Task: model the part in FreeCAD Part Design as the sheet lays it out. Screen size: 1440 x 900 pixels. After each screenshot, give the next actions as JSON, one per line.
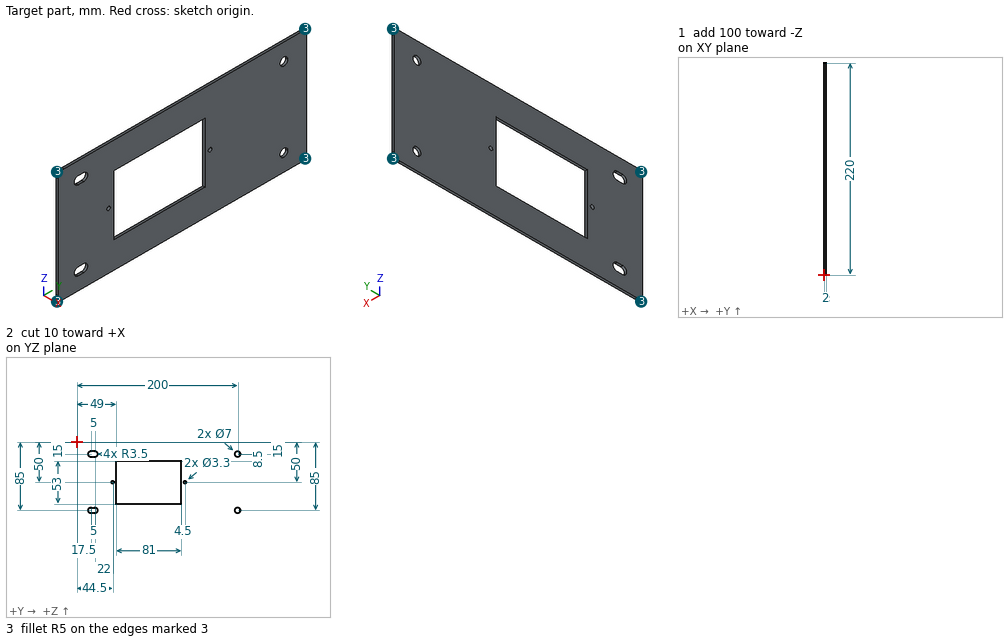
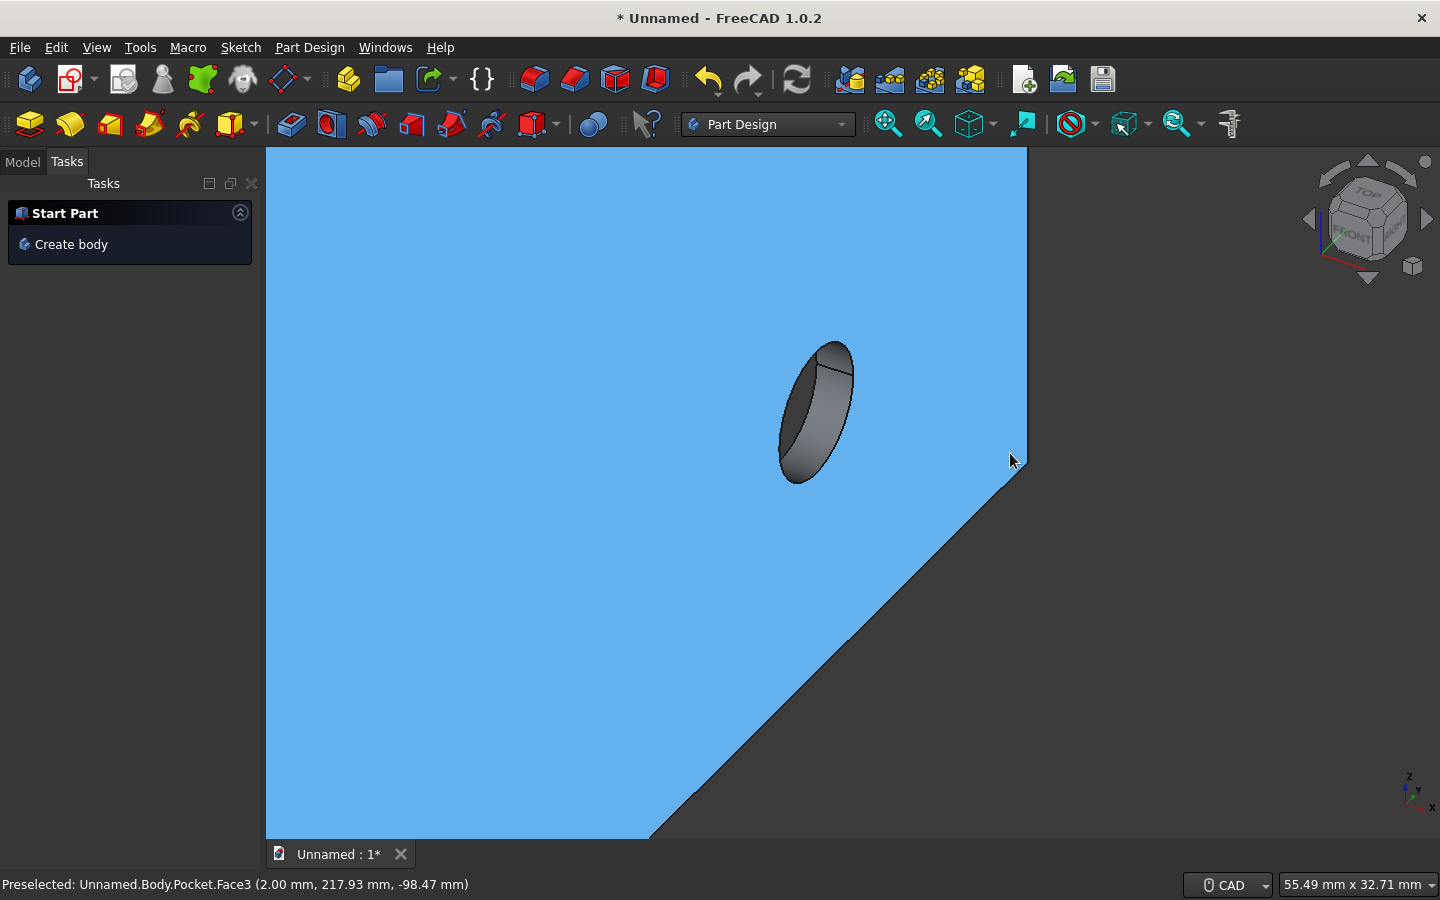
{"action": "left_click", "coordinate": [890, 124]}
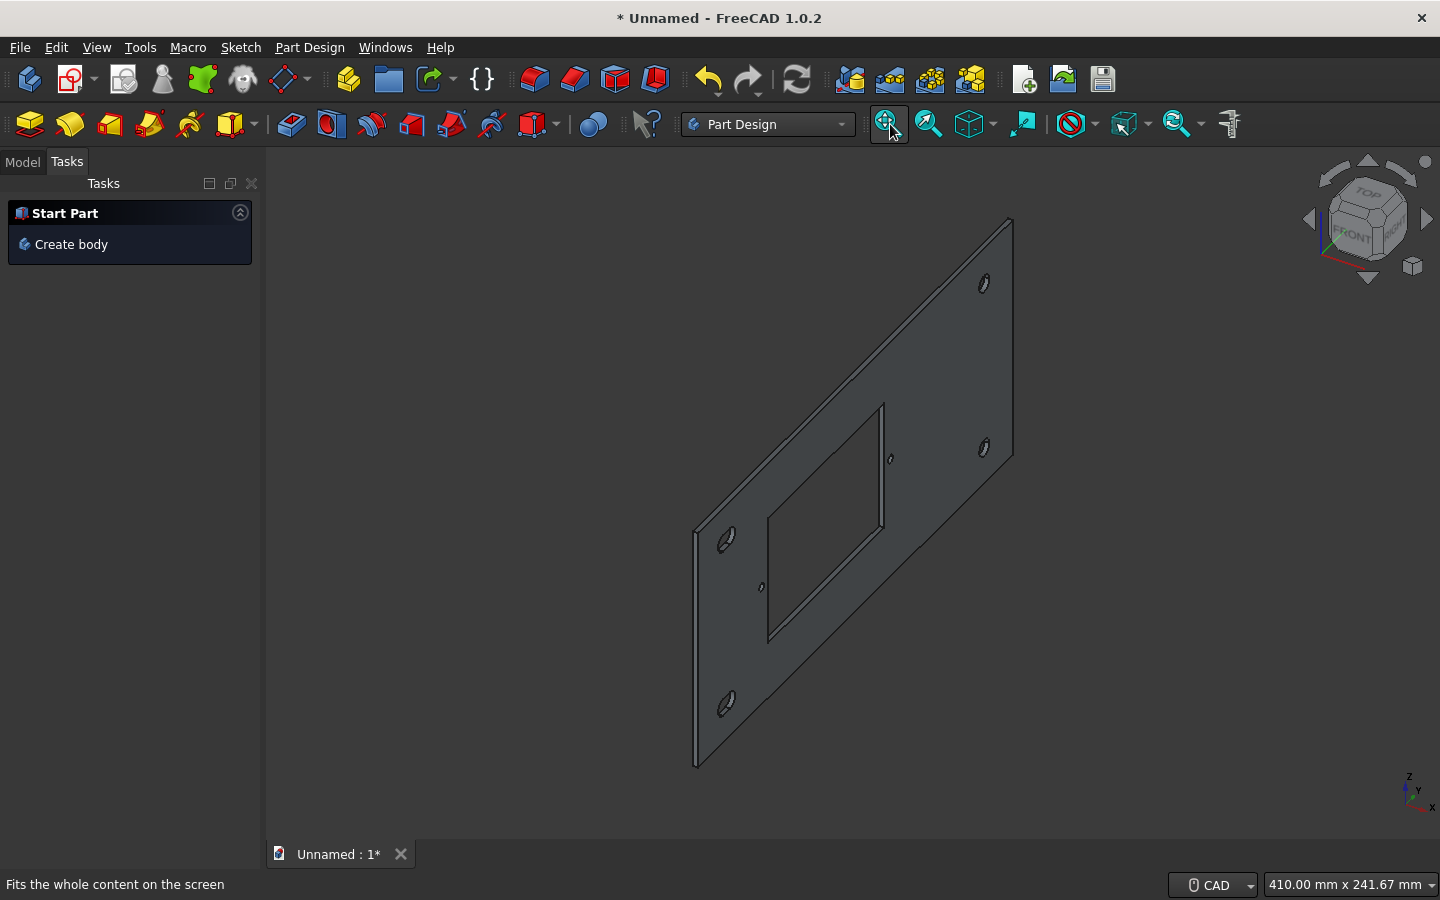
{"action": "key", "text": "0"}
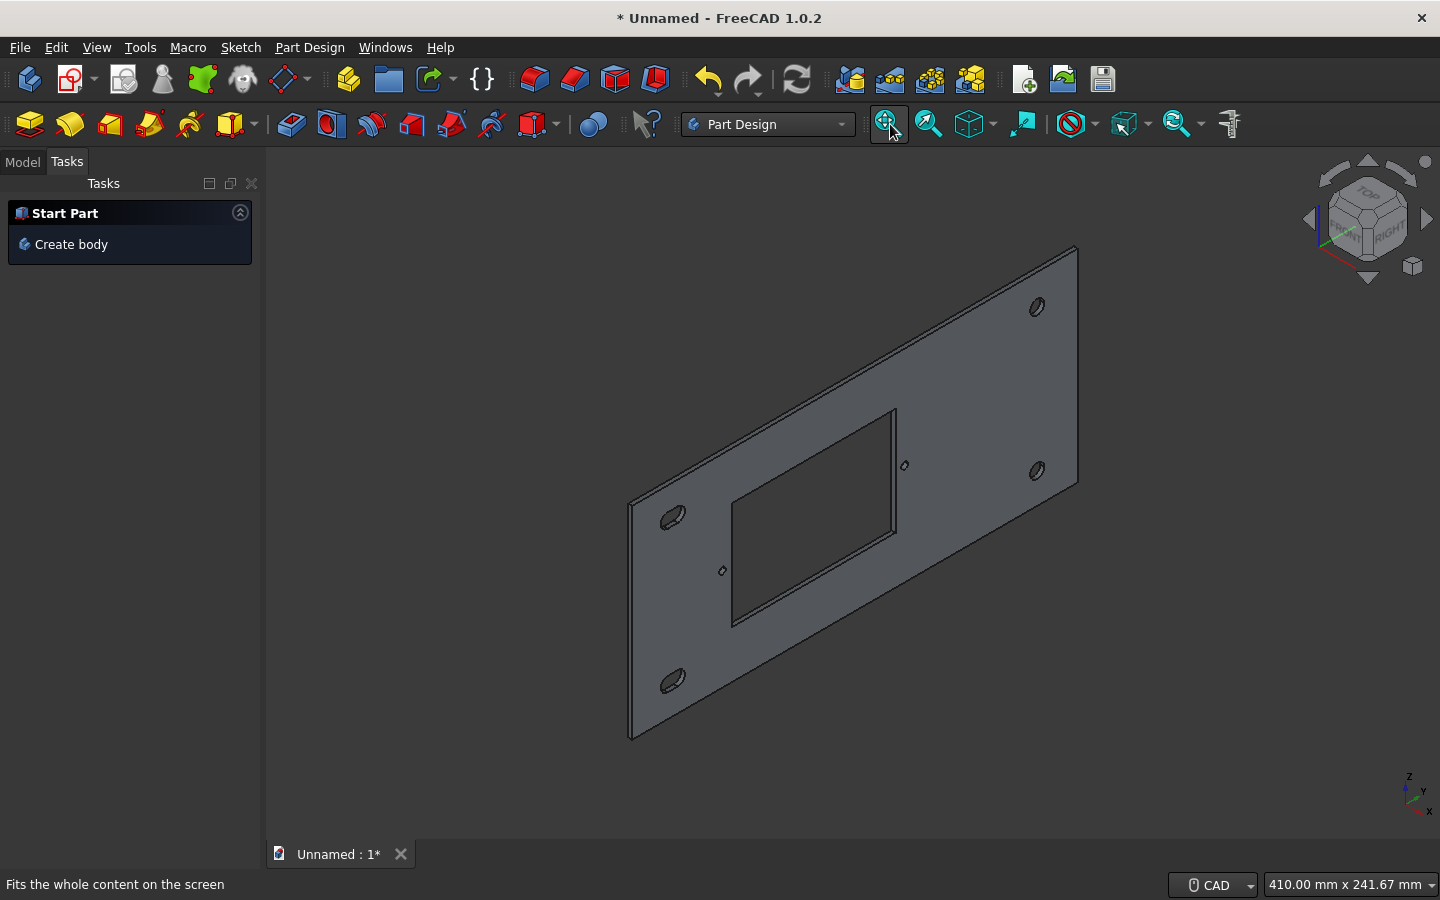
{"action": "scroll", "coordinate": [1076, 480], "scroll_direction": "up", "scroll_amount": 10}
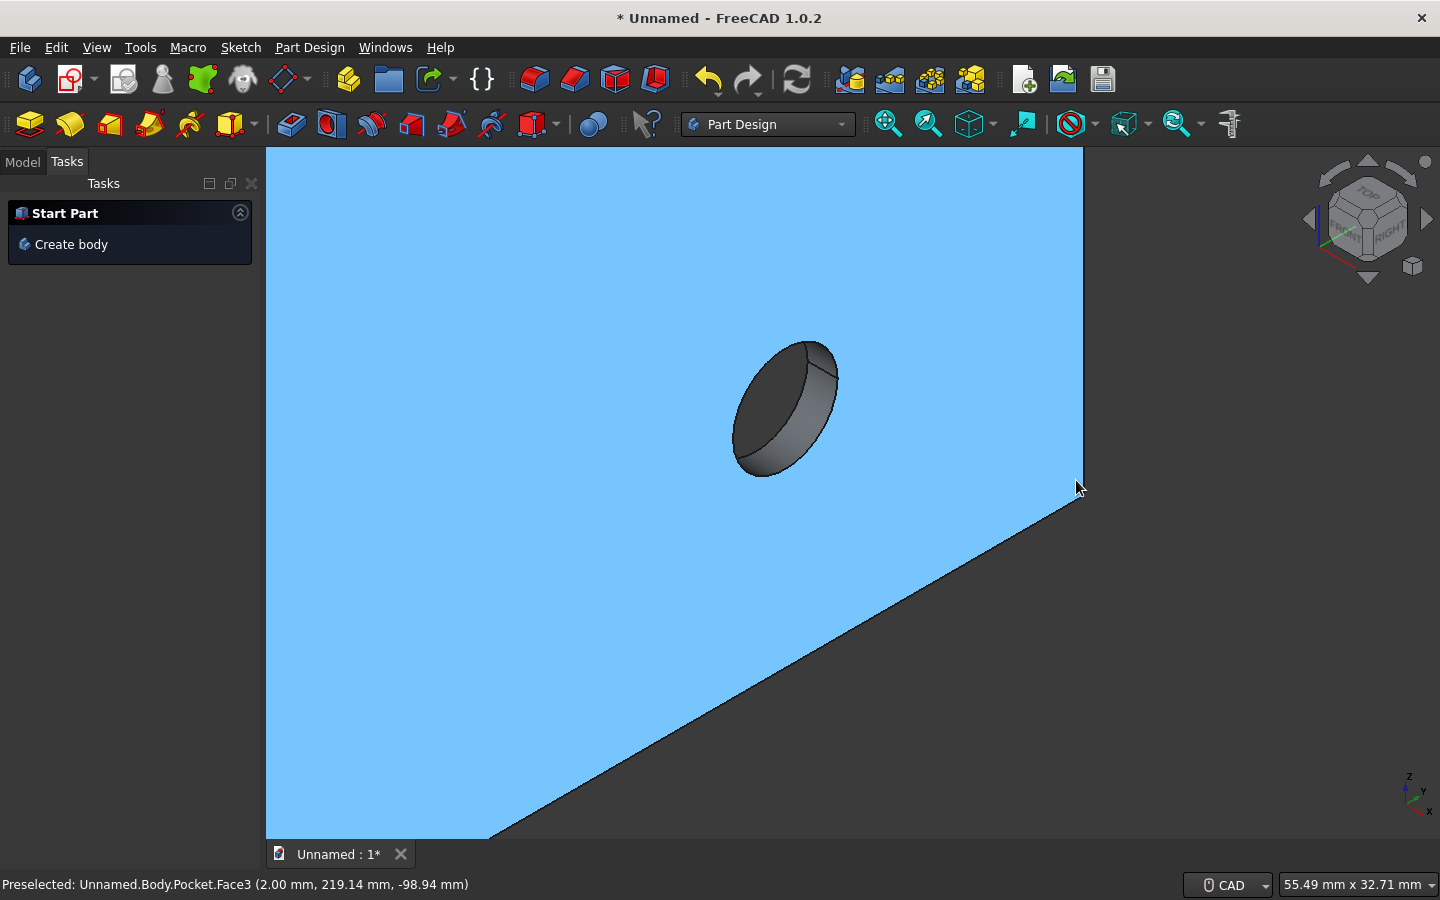
{"action": "left_click", "coordinate": [890, 124]}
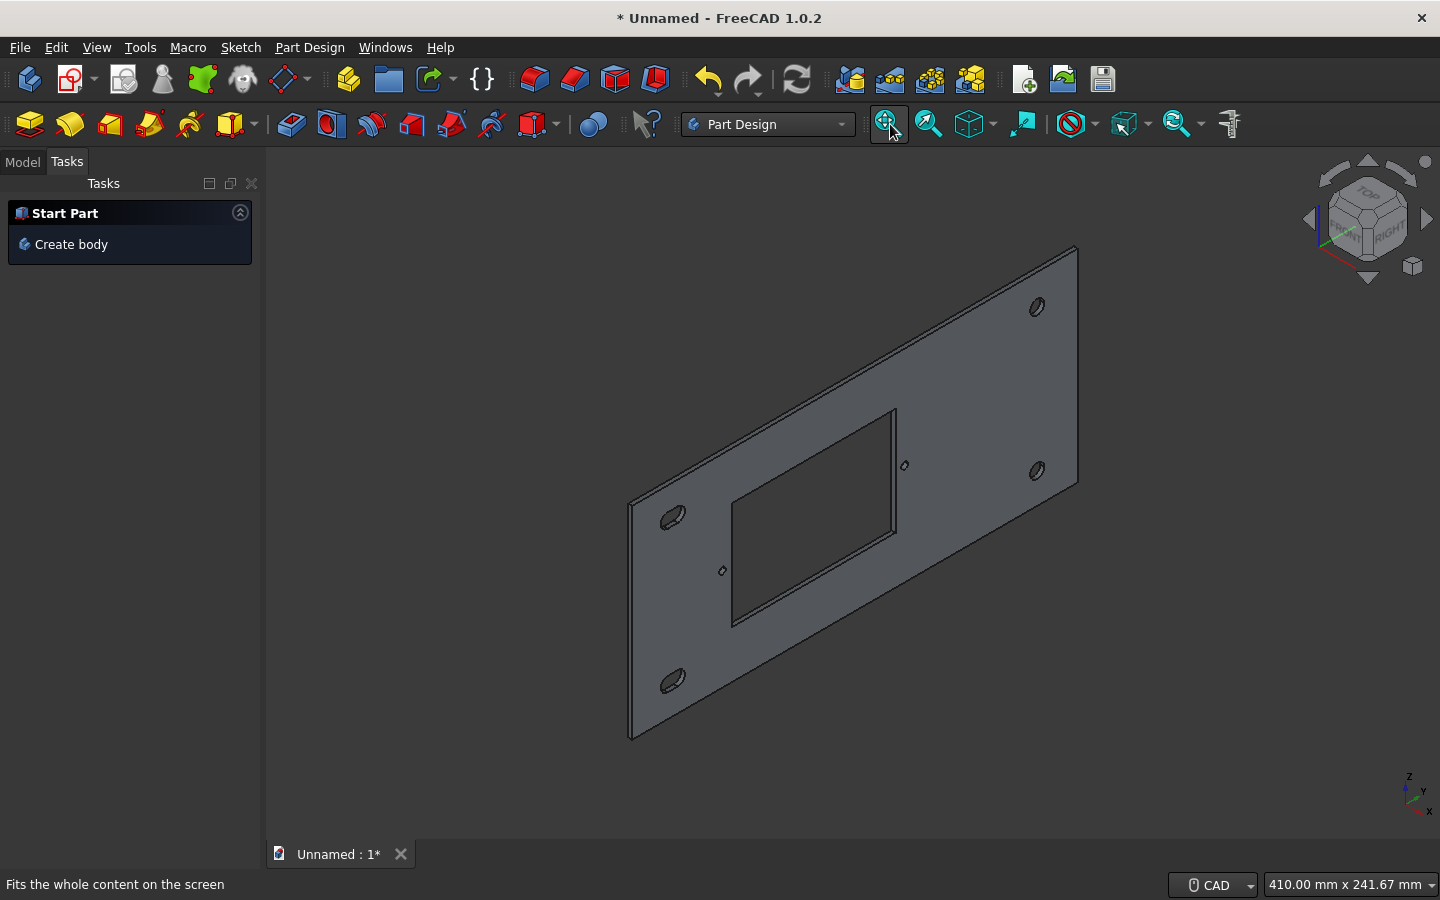
{"action": "key", "text": "2"}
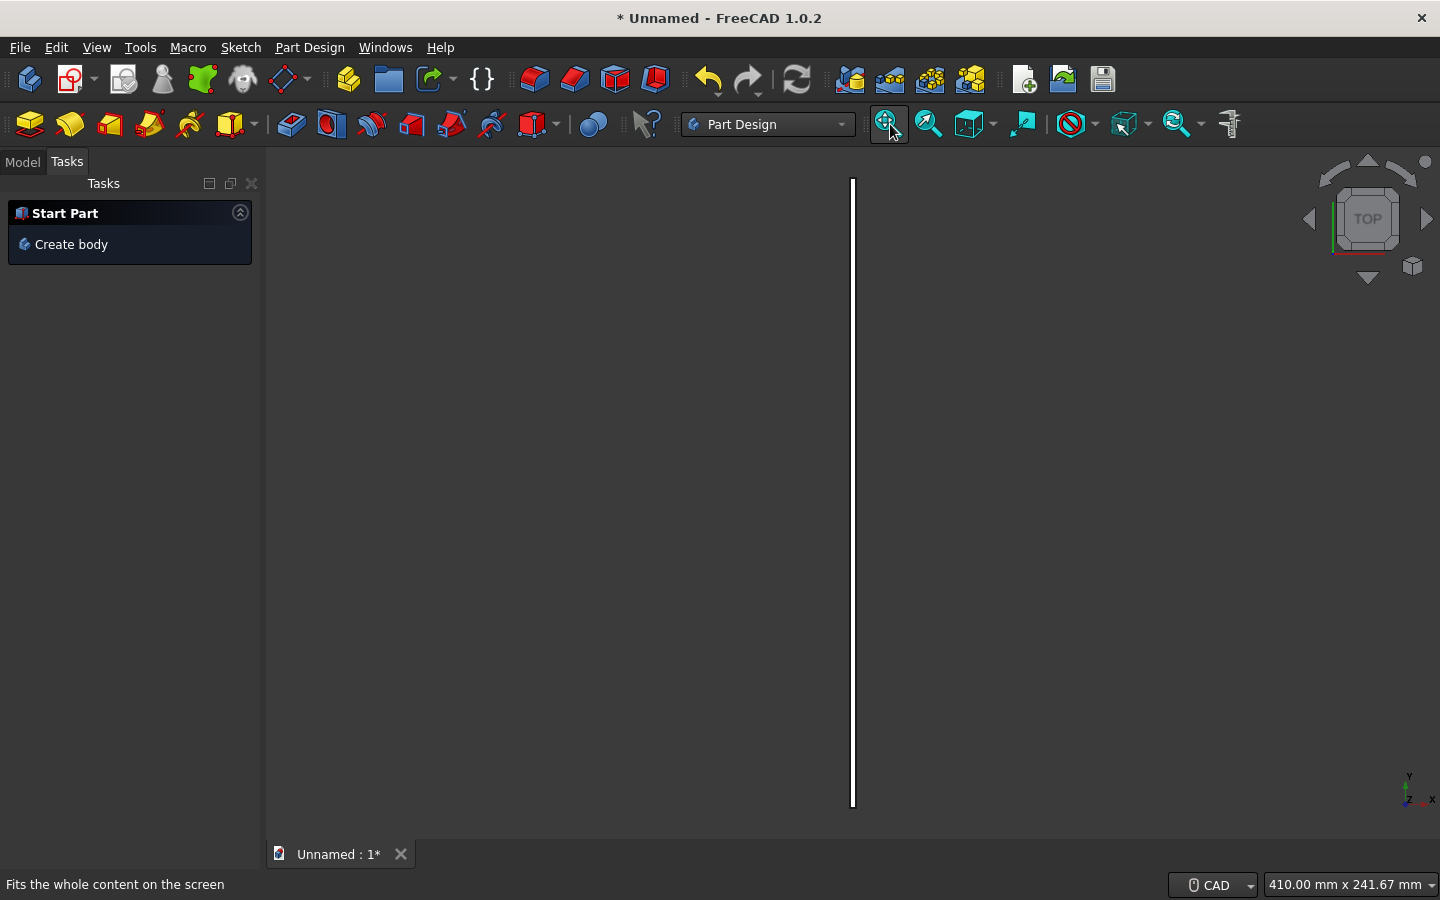
{"action": "scroll", "coordinate": [853, 177], "scroll_direction": "up", "scroll_amount": 10}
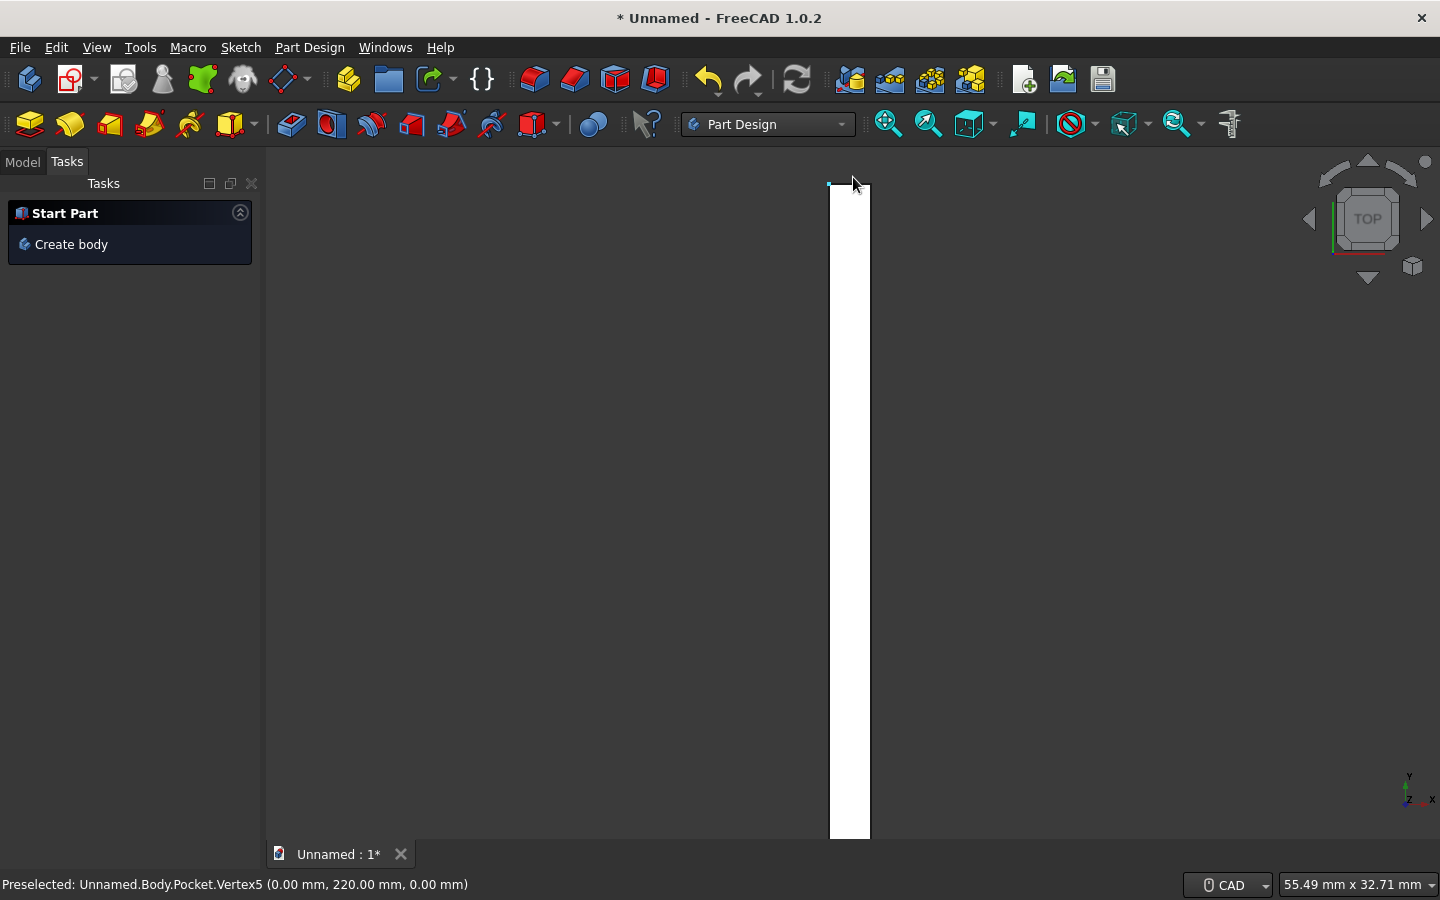
{"action": "left_click", "coordinate": [850, 183]}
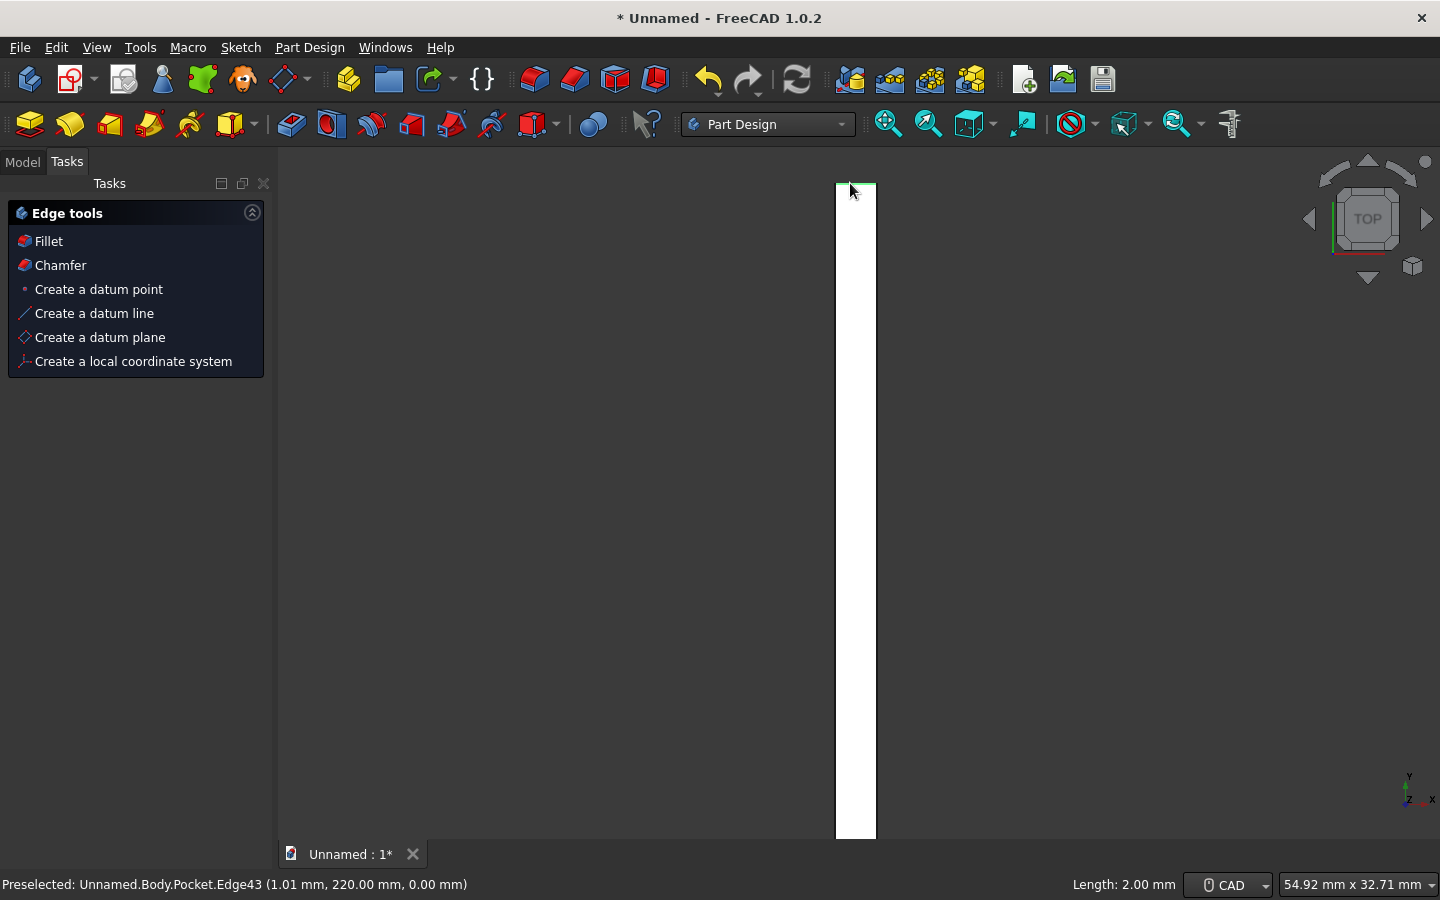
{"action": "left_click", "coordinate": [890, 124]}